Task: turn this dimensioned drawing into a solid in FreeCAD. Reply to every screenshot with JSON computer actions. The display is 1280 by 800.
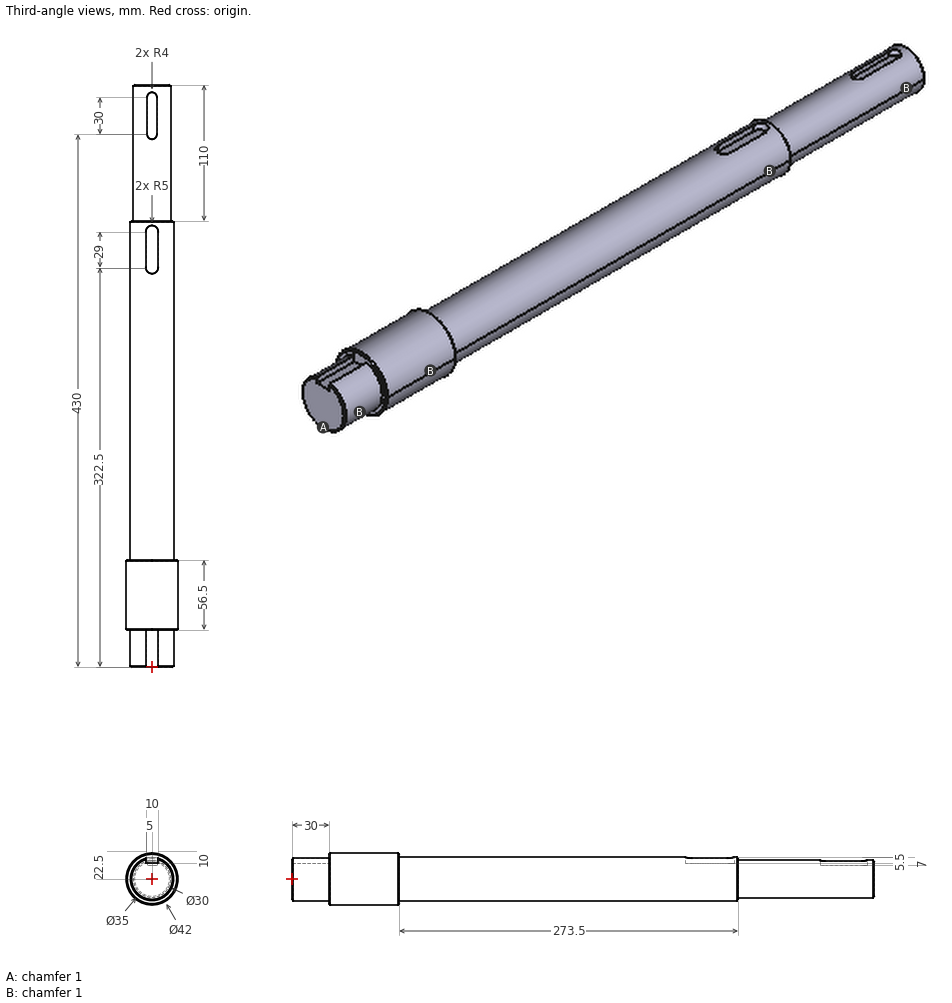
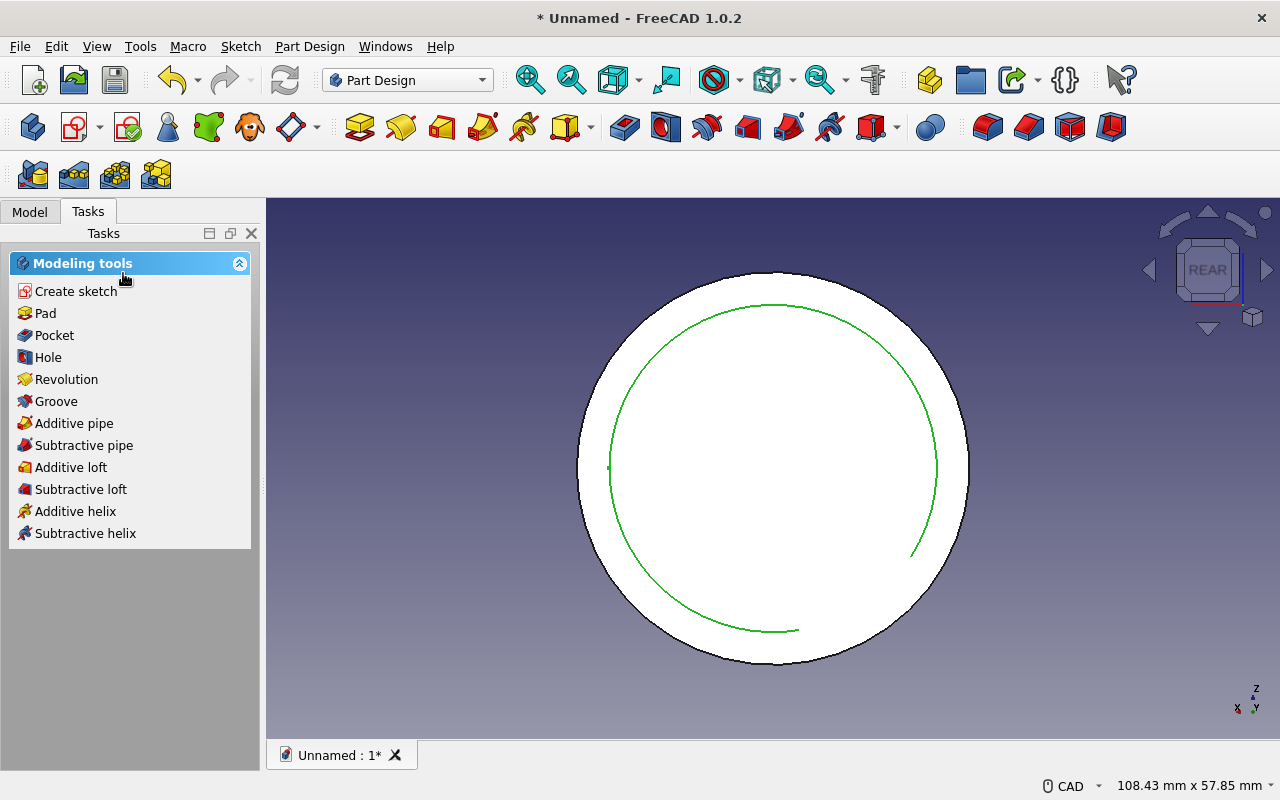
{"action": "left_click", "coordinate": [360, 128]}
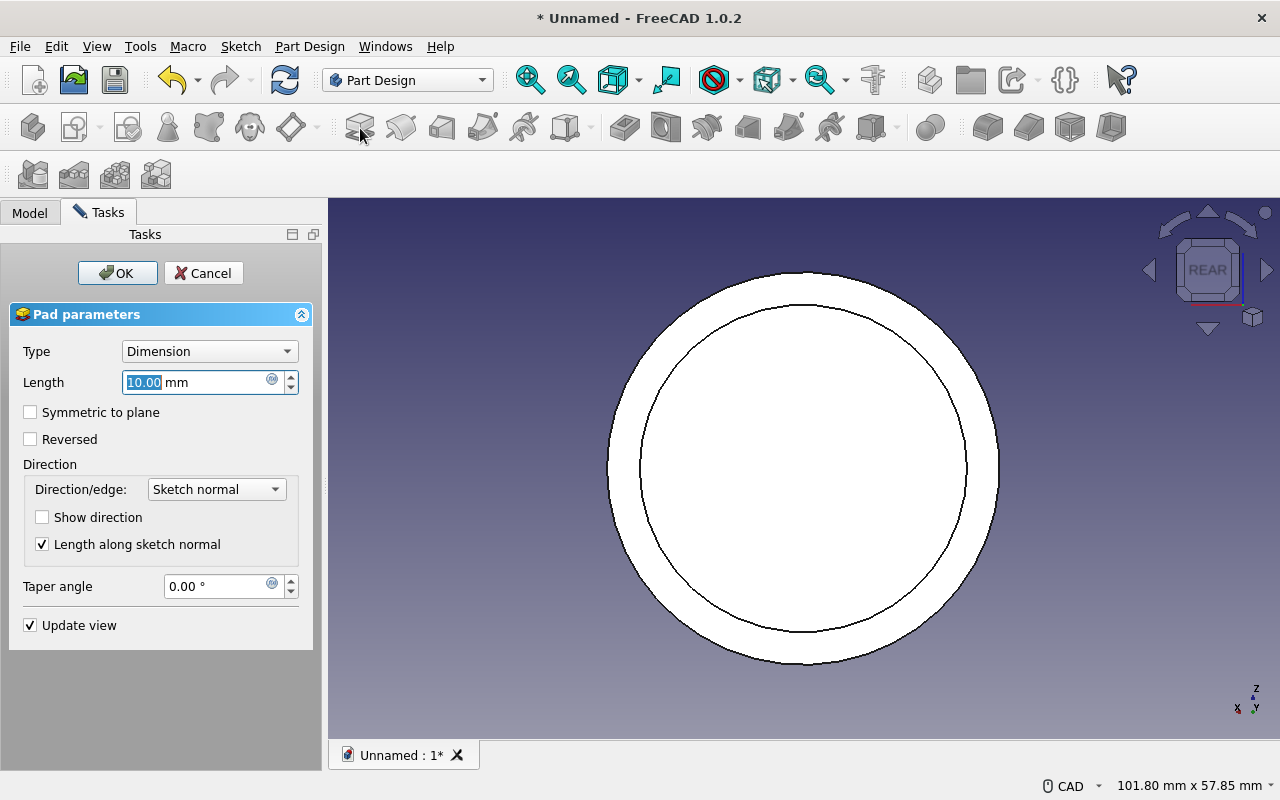
{"action": "type", "text": "273.5"}
{"action": "key", "text": "Tab"}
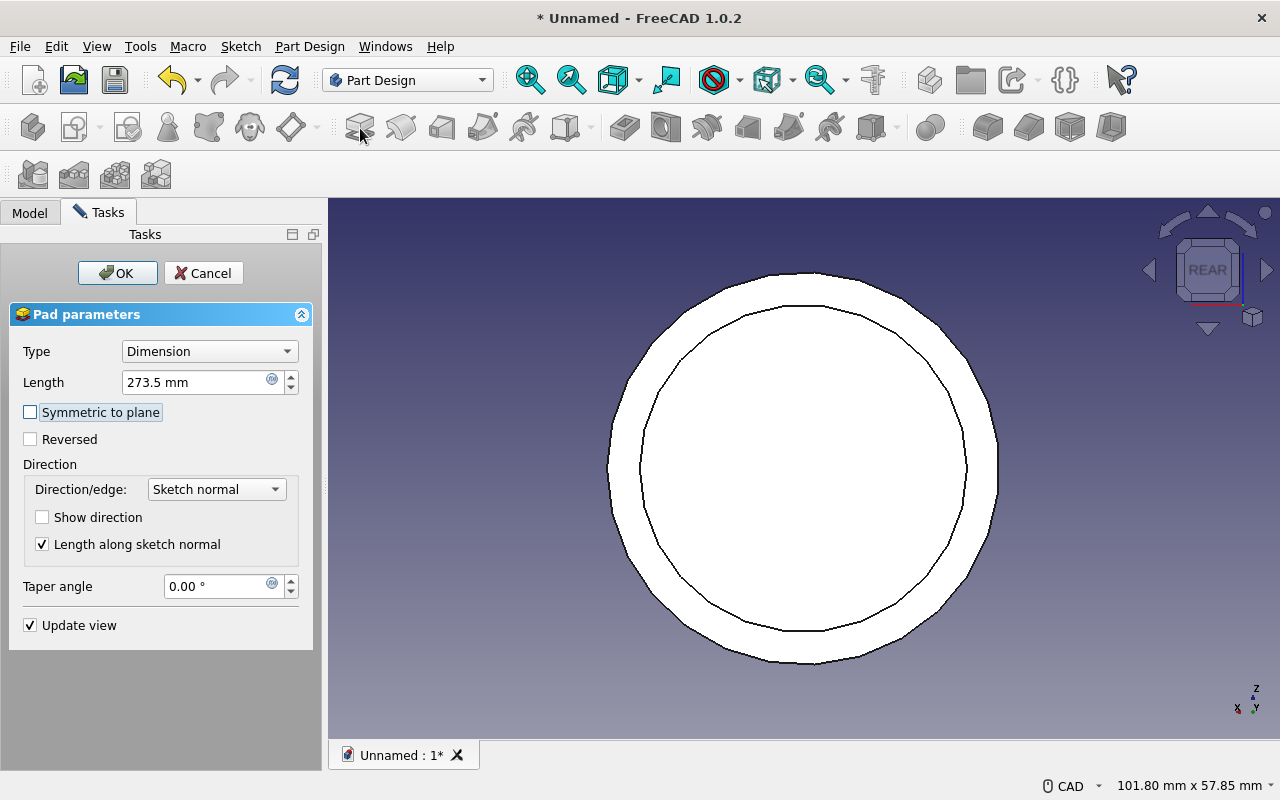
{"action": "left_click", "coordinate": [118, 273]}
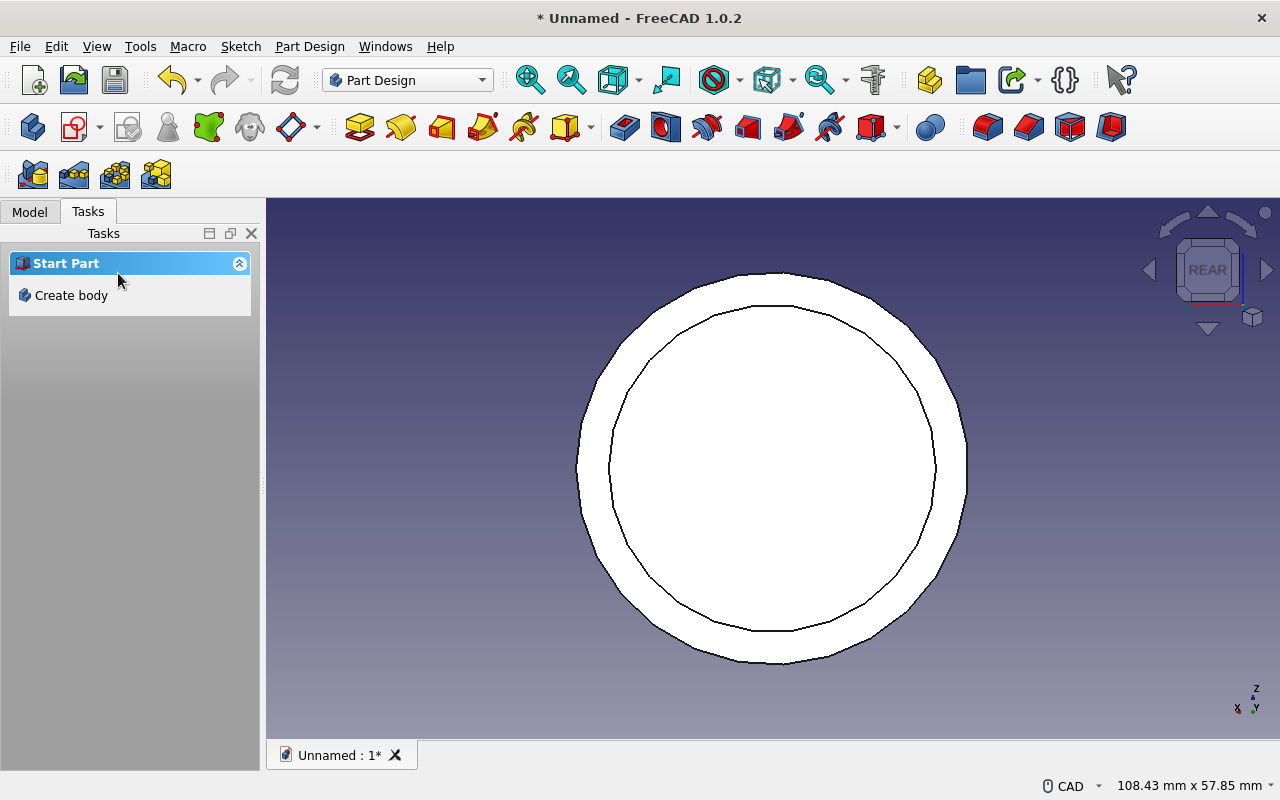
{"action": "left_click", "coordinate": [772, 467]}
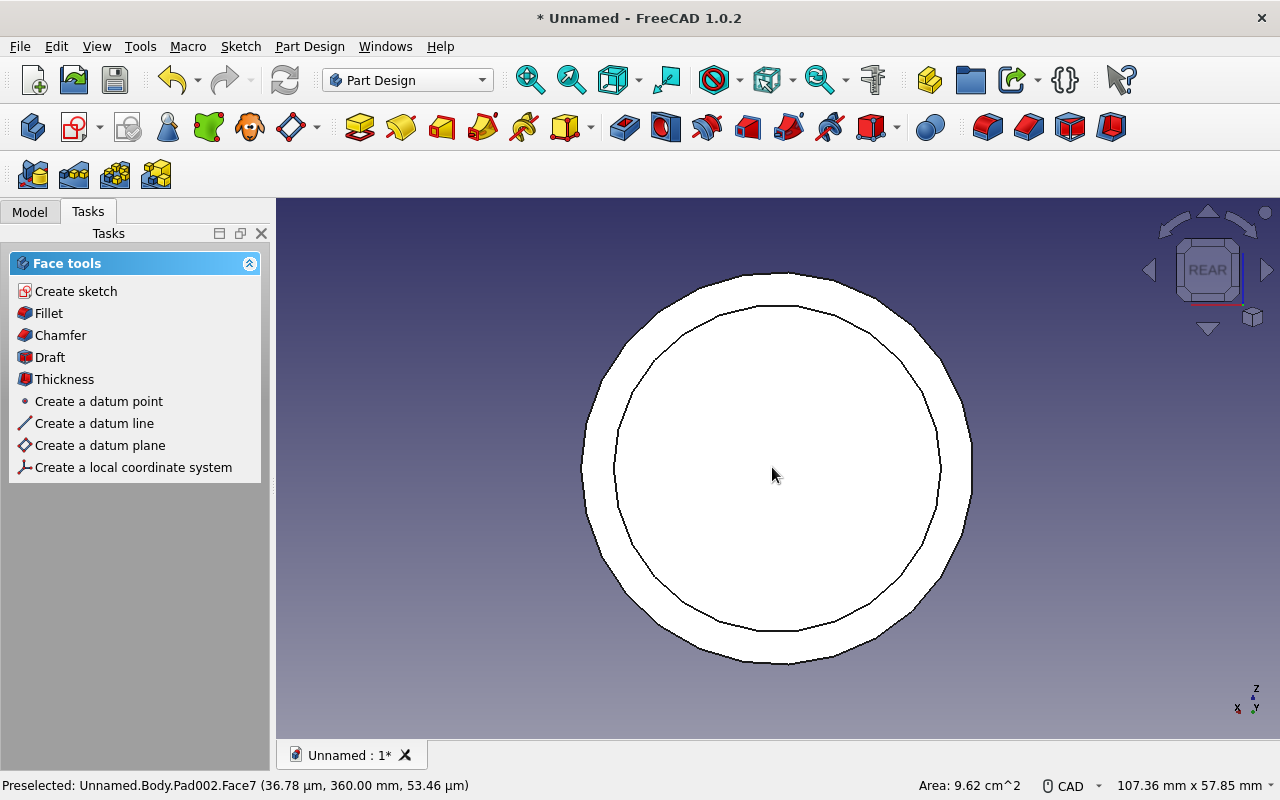
{"action": "left_click", "coordinate": [74, 128]}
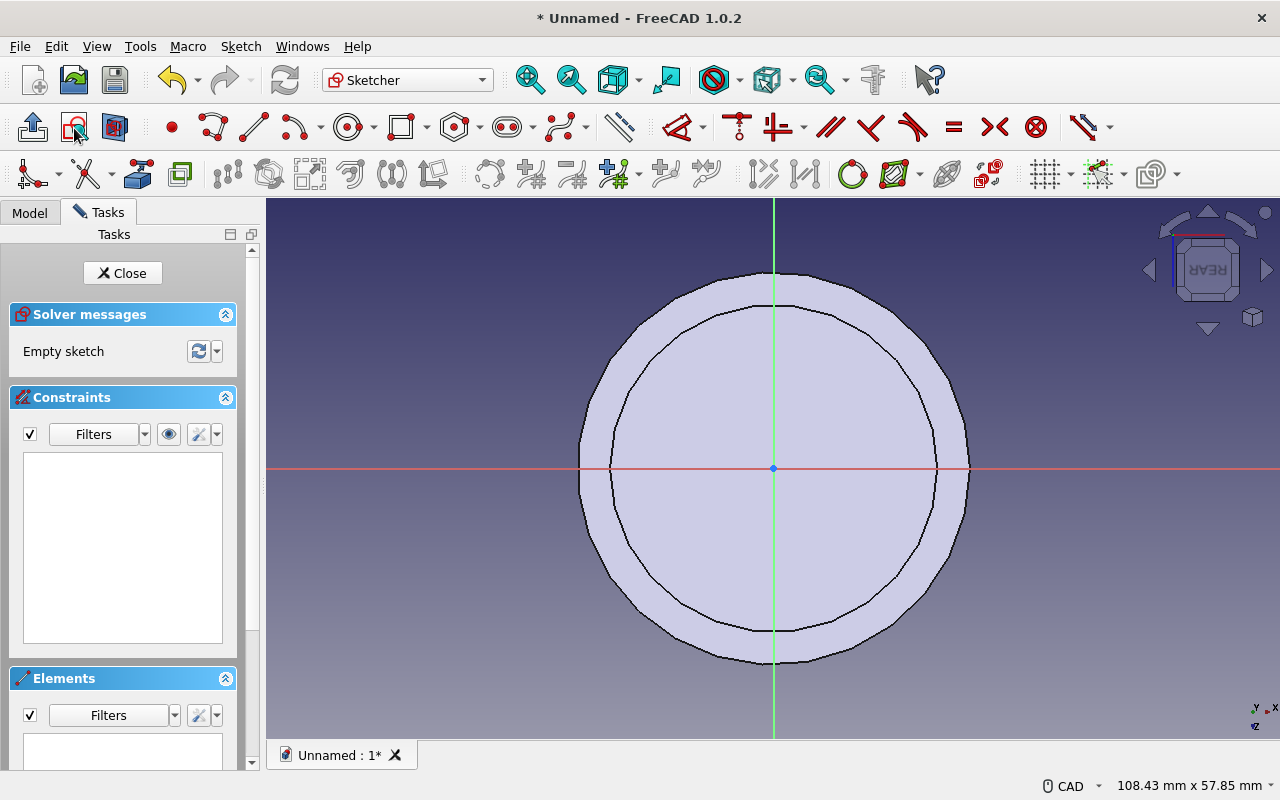
{"action": "key", "text": "g c"}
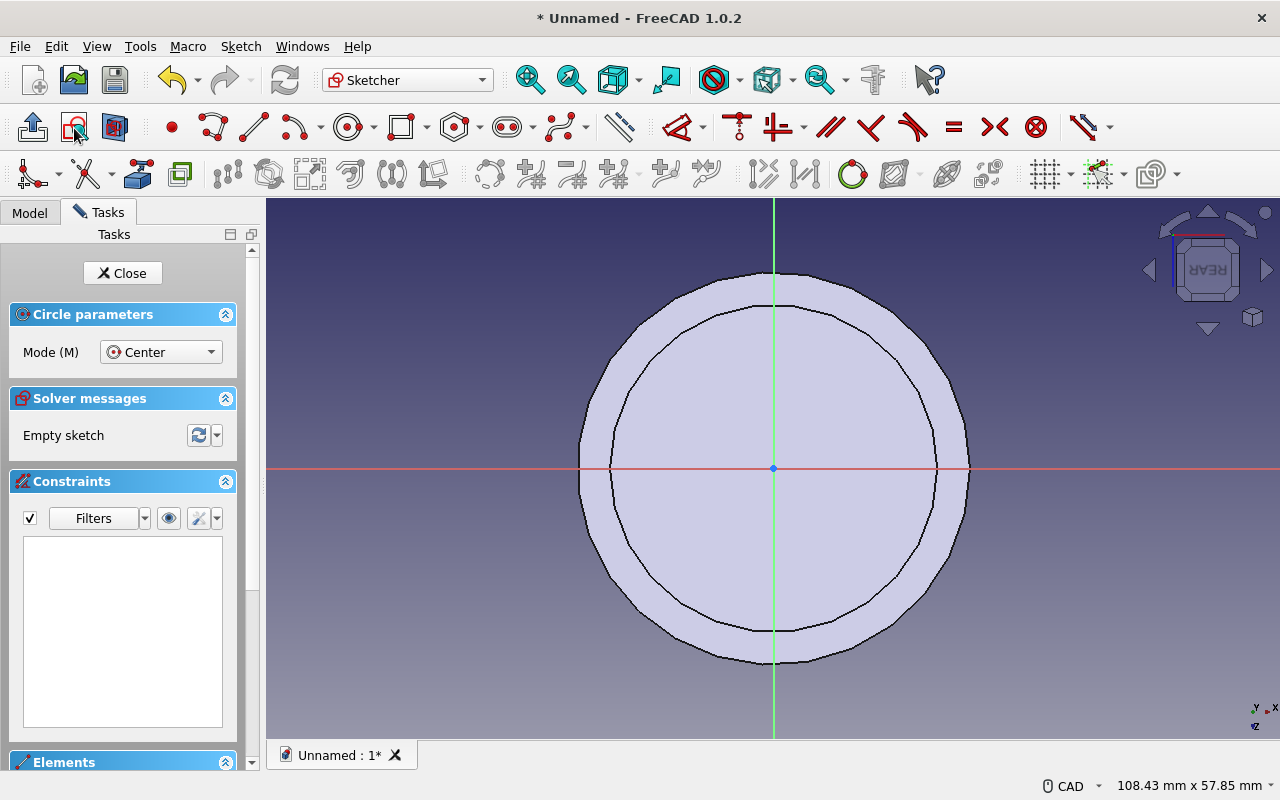
{"action": "left_click", "coordinate": [774, 468]}
{"action": "mouse_move", "coordinate": [873, 369]}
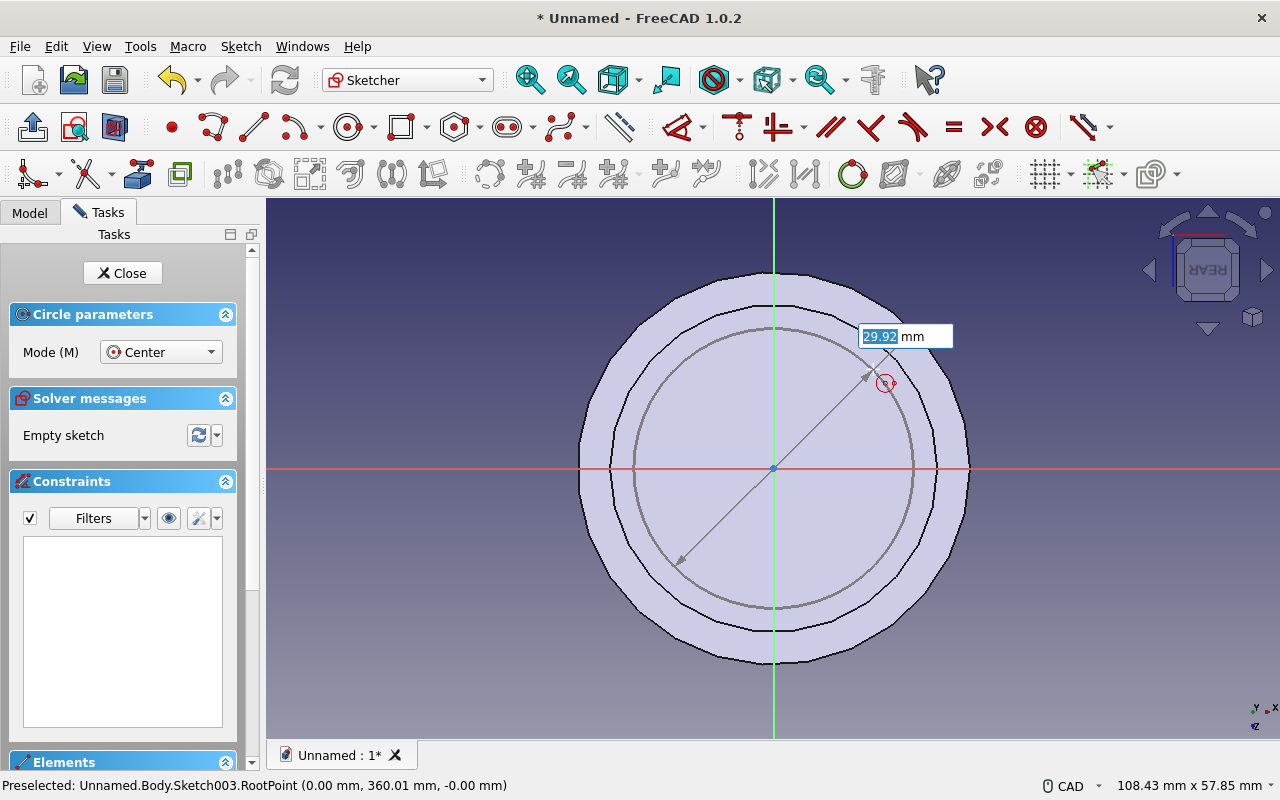
{"action": "type", "text": "30"}
{"action": "key", "text": "Return"}
{"action": "key", "text": "Escape"}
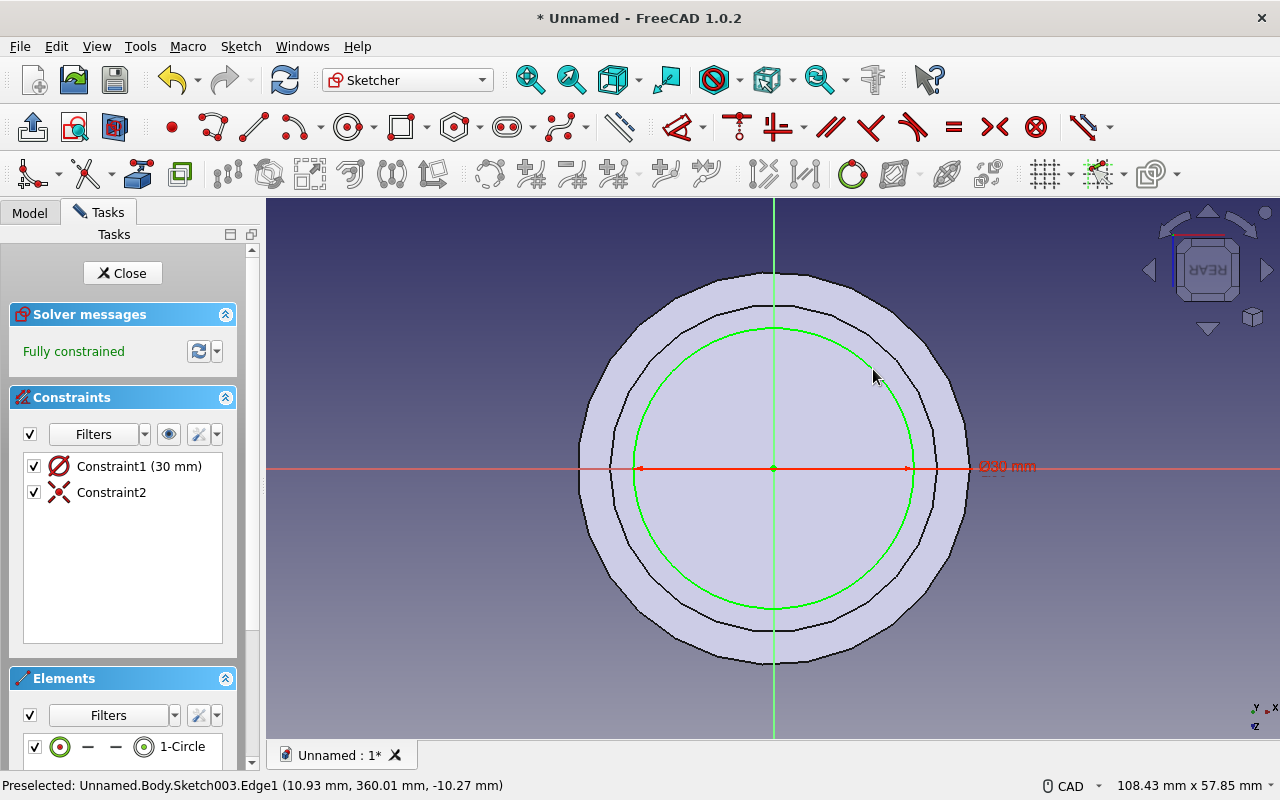
{"action": "left_click", "coordinate": [123, 273]}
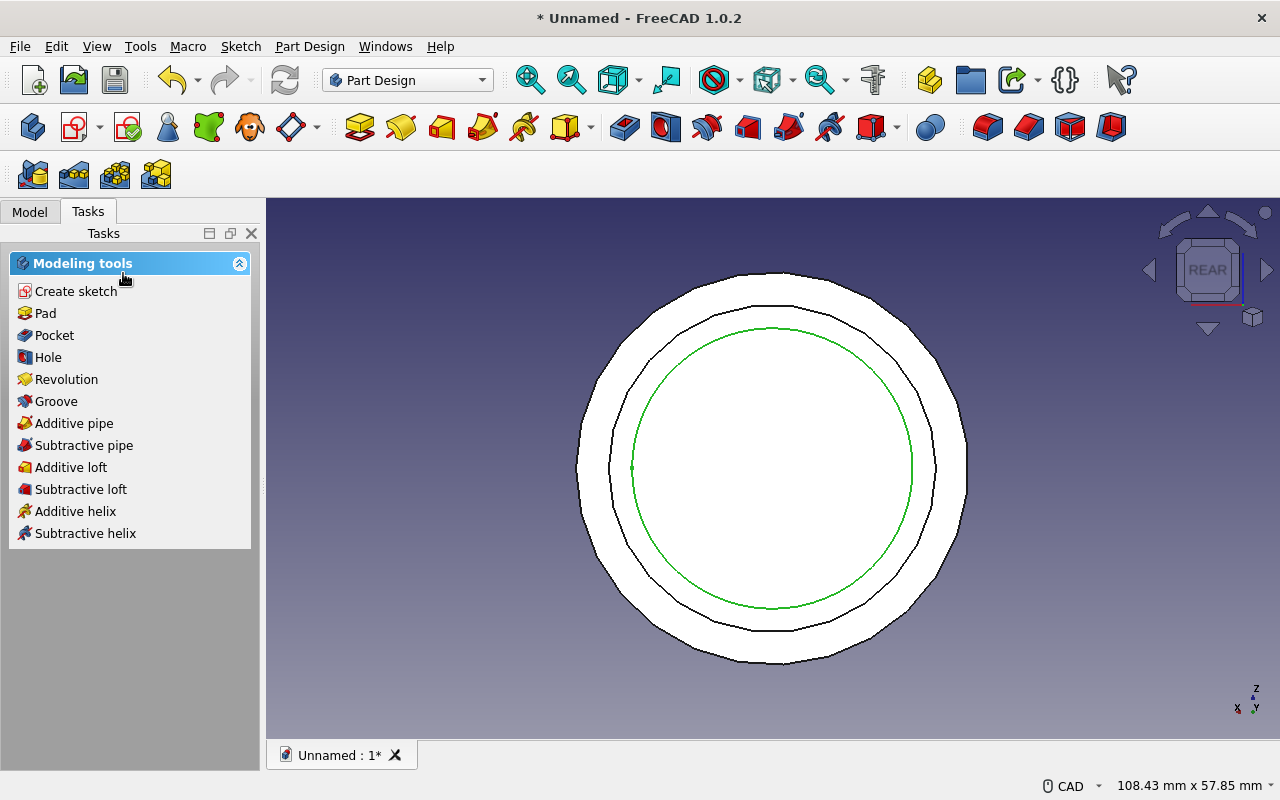
{"action": "left_click", "coordinate": [360, 128]}